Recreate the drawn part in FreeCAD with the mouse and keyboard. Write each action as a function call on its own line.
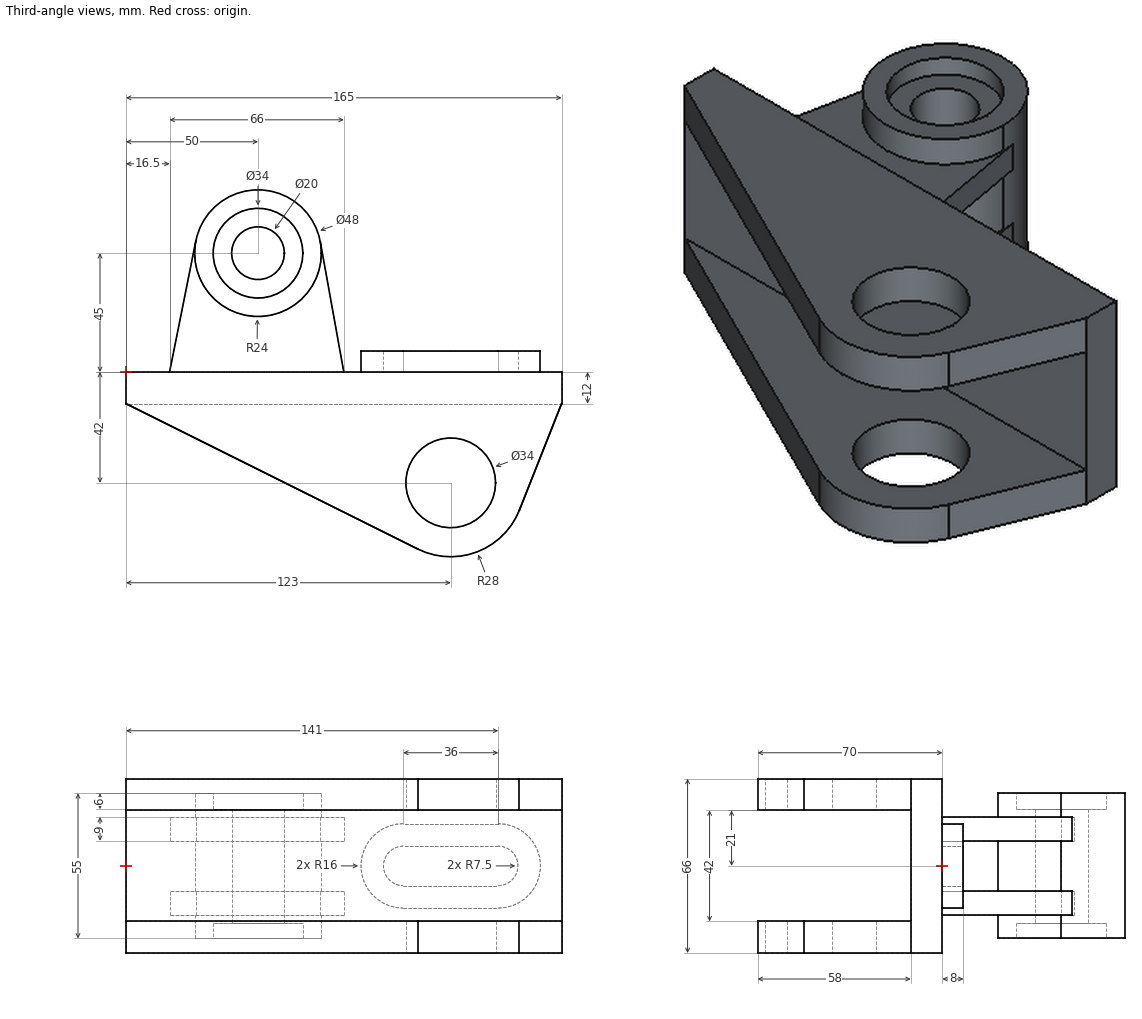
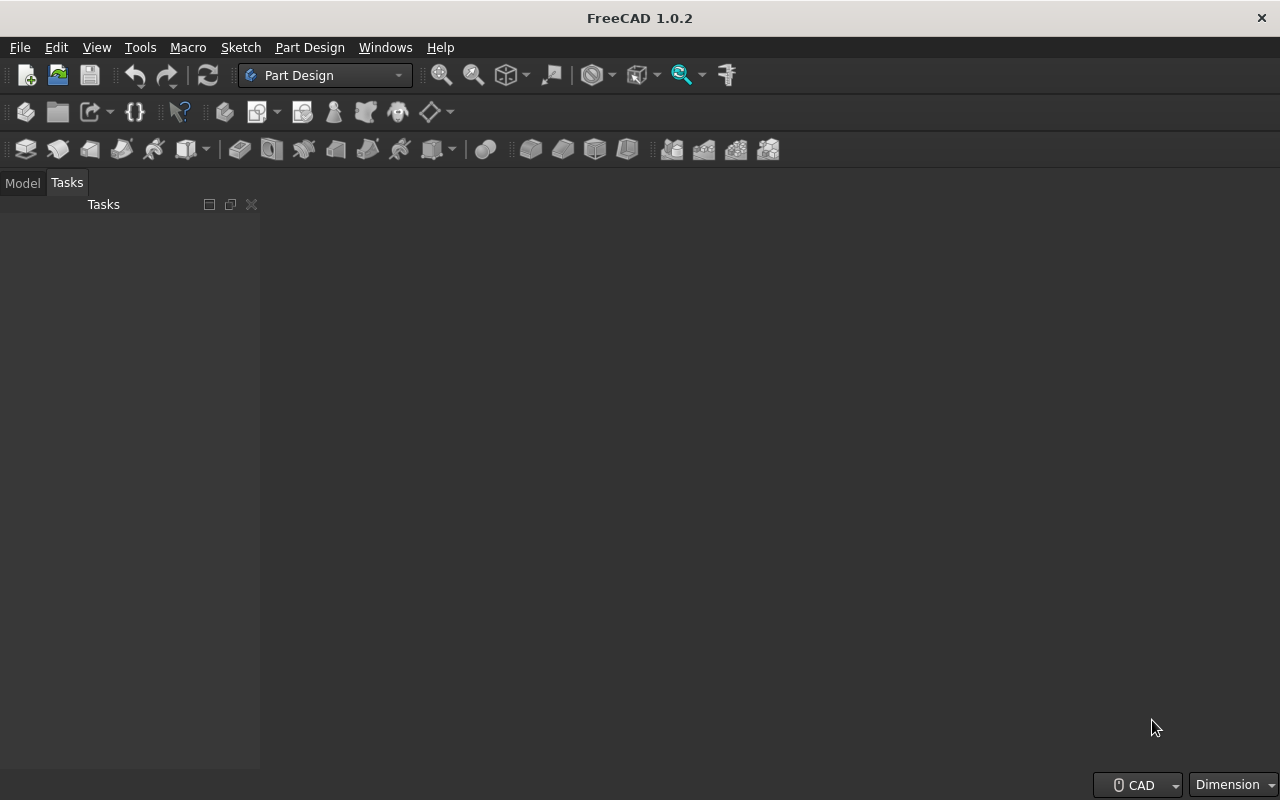
key(ctrl+n)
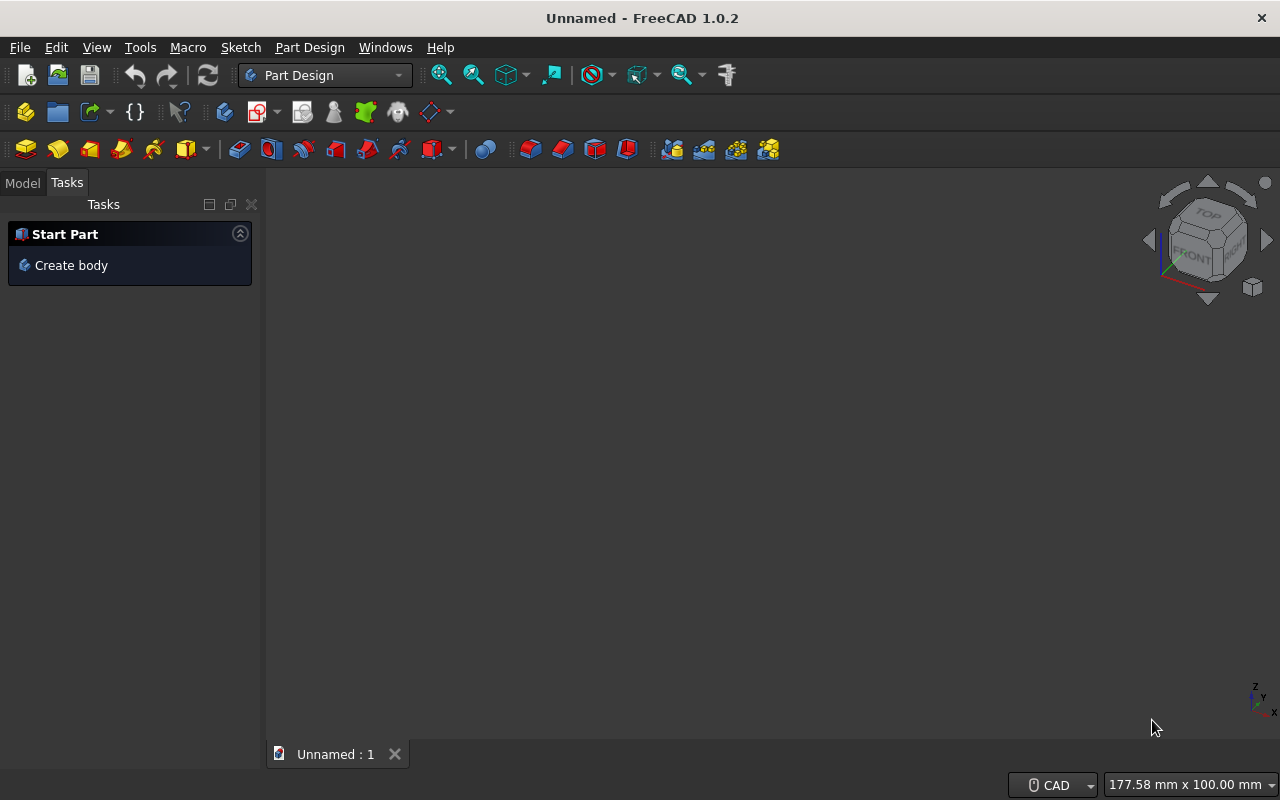
click(258, 112)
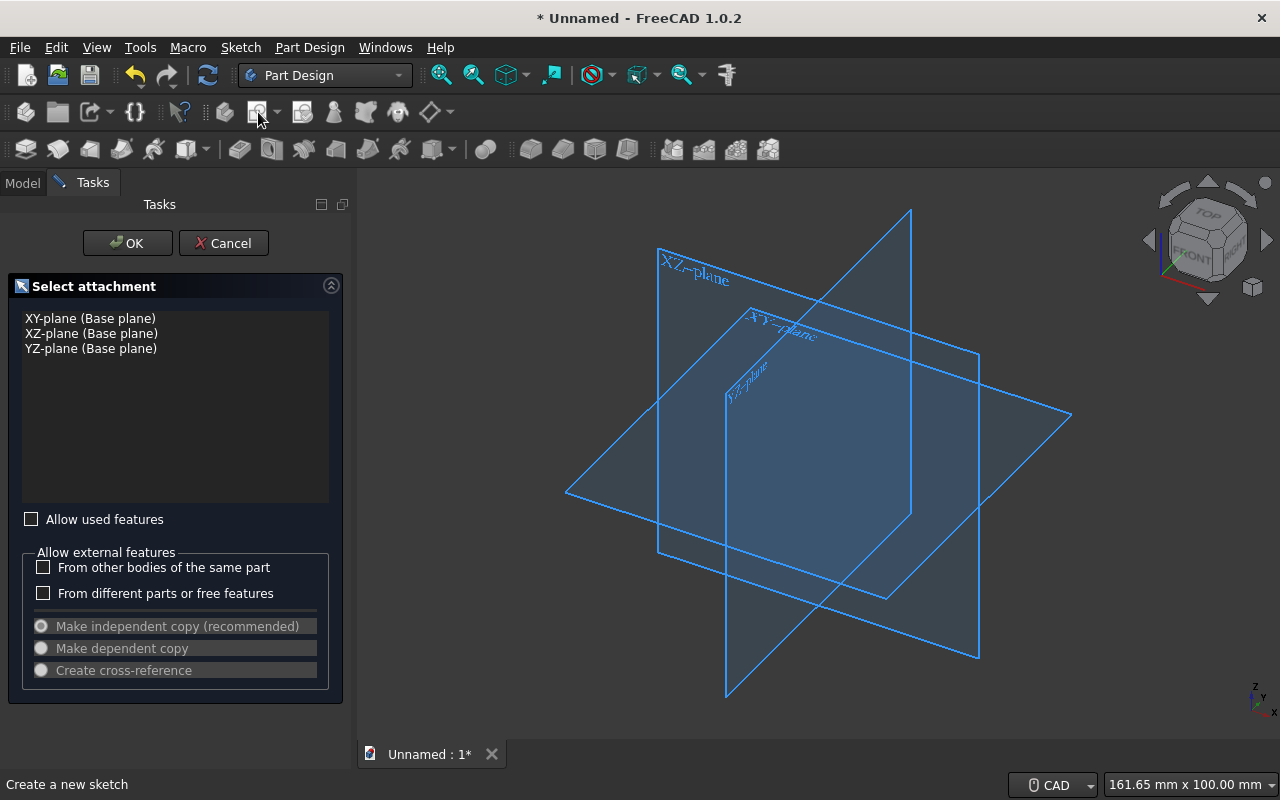
click(82, 318)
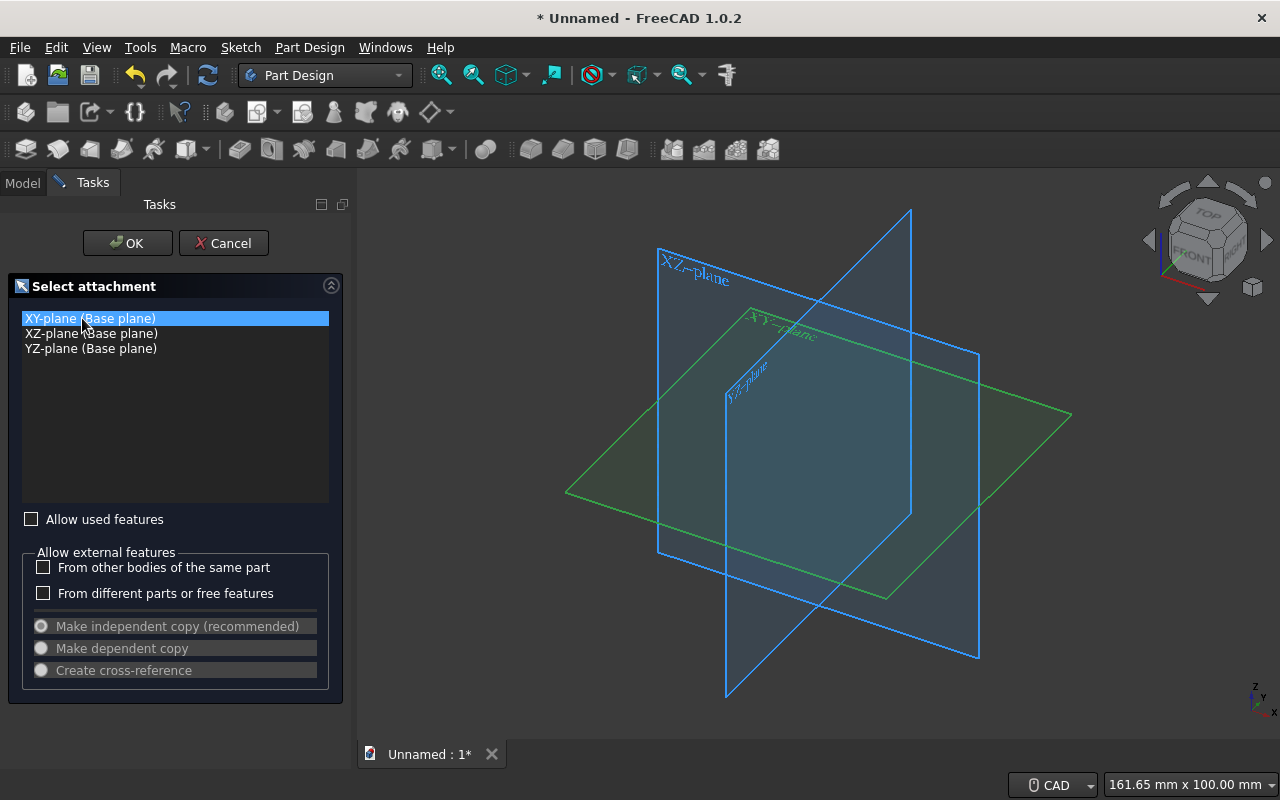
click(128, 243)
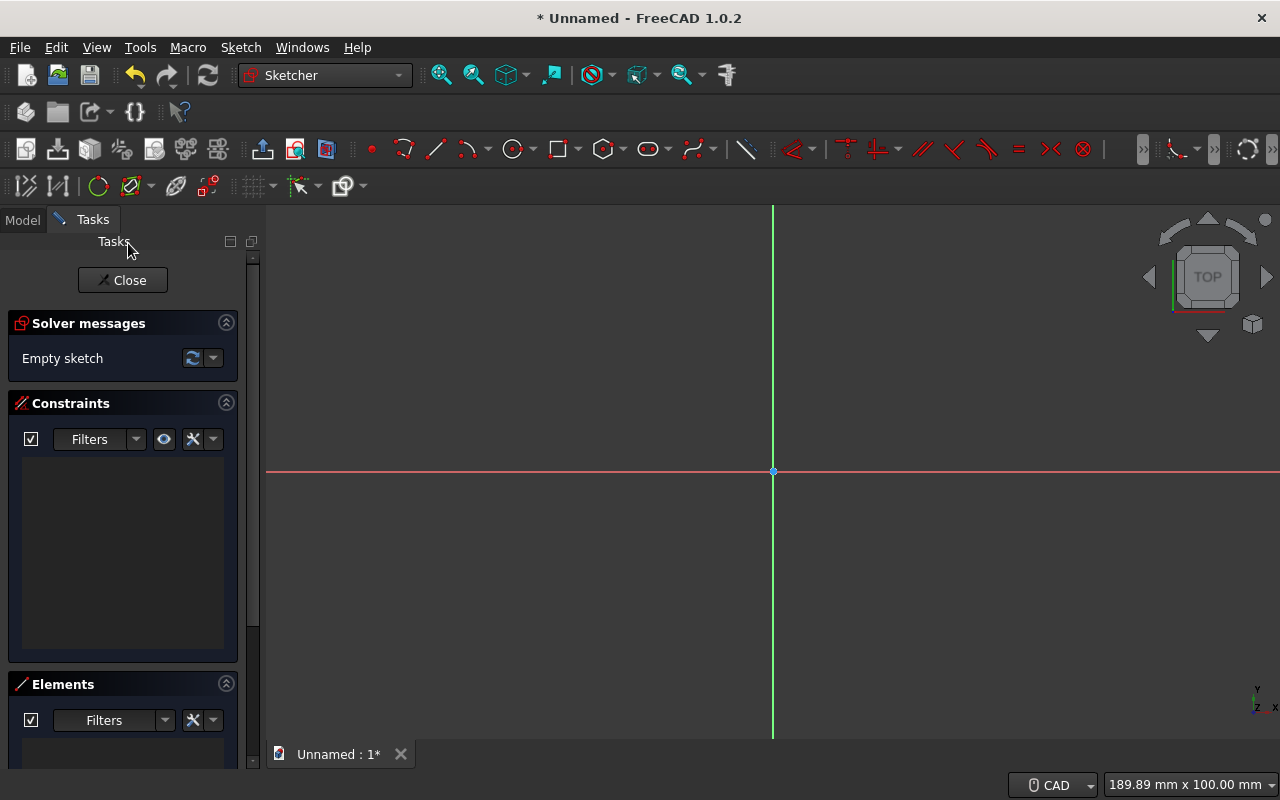
scroll(294, 251, down, 3)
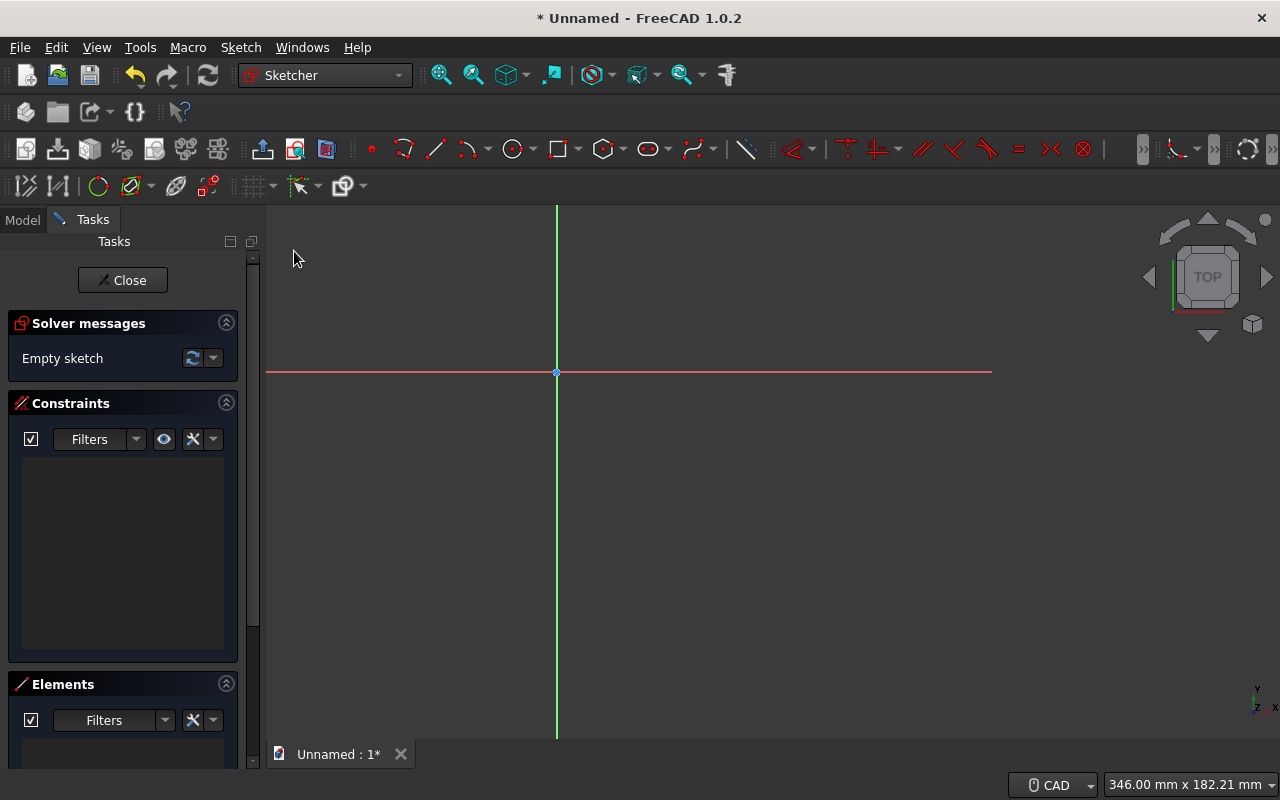
key(g)
key(m)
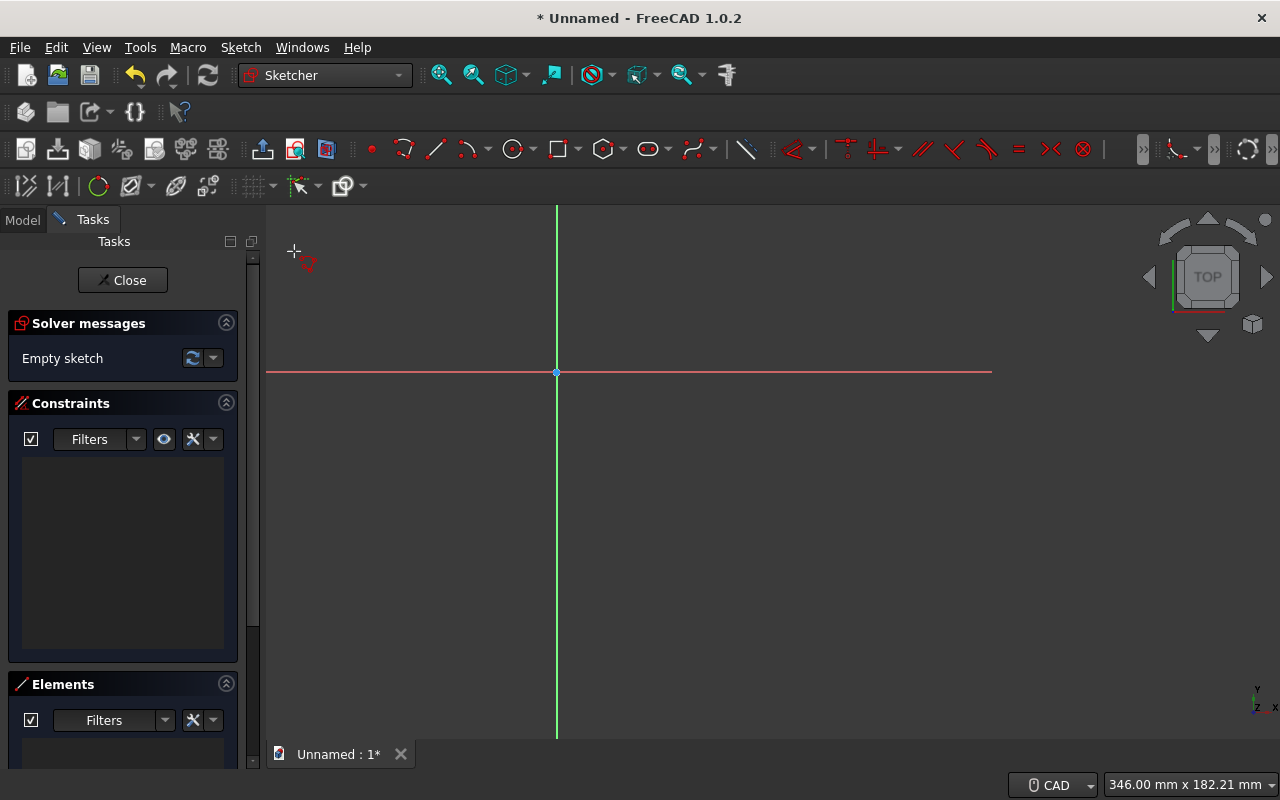
click(994, 526)
click(1040, 407)
click(1040, 372)
click(557, 372)
click(566, 407)
click(881, 569)
right_click(881, 569)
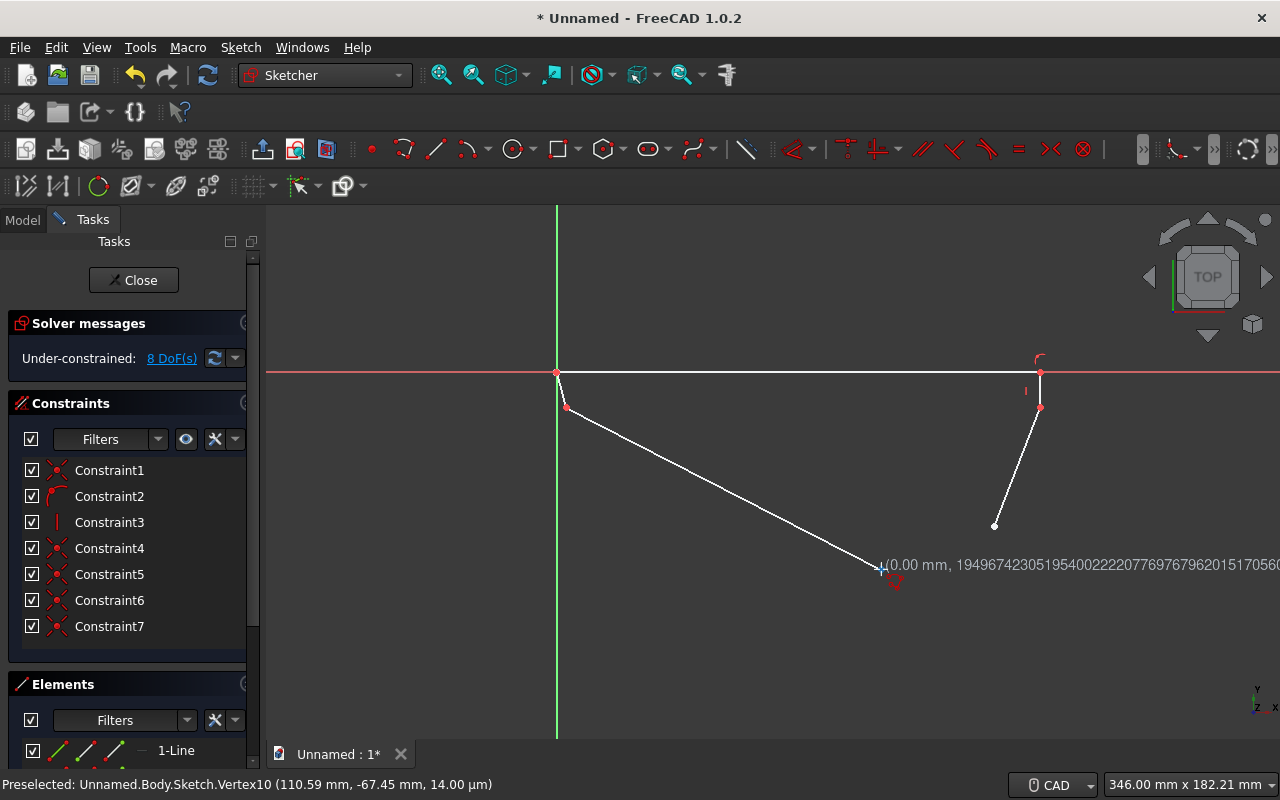
key(g)
key(3)
key(a)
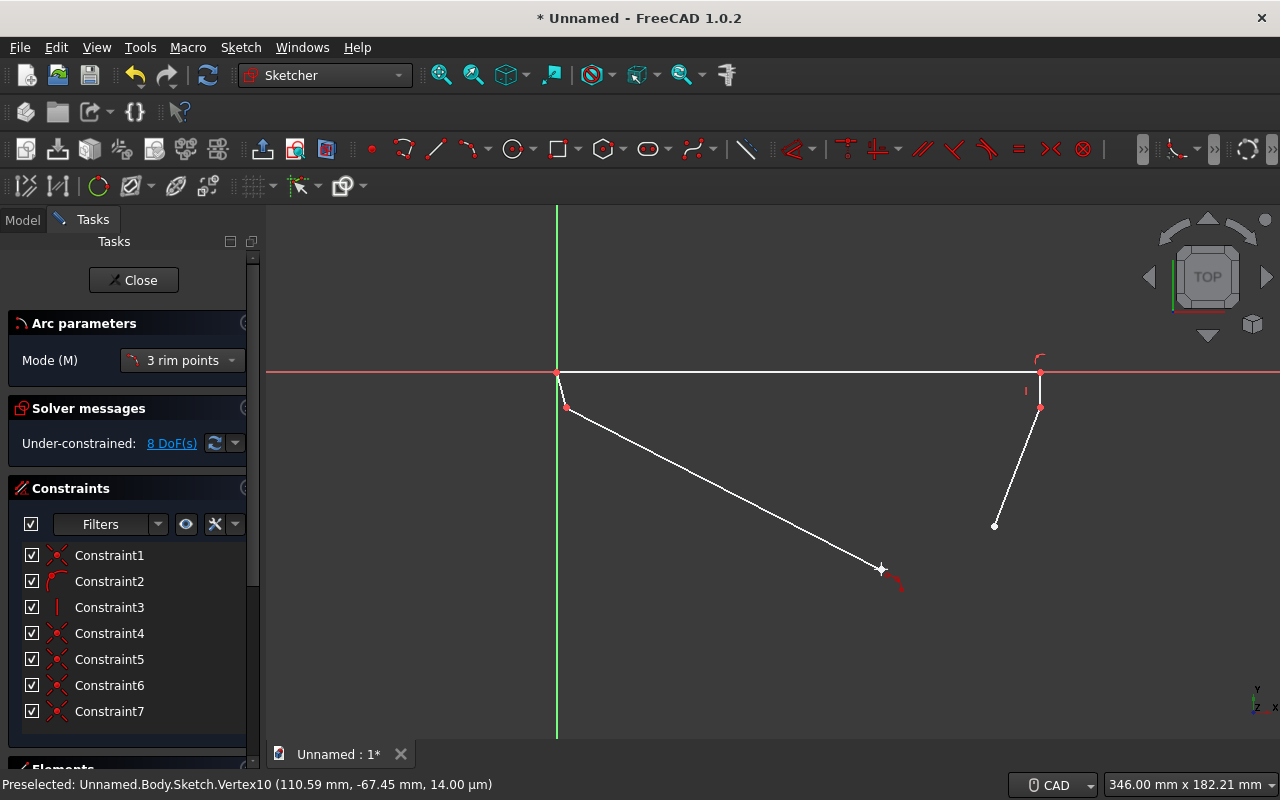
click(881, 570)
click(994, 527)
click(947, 572)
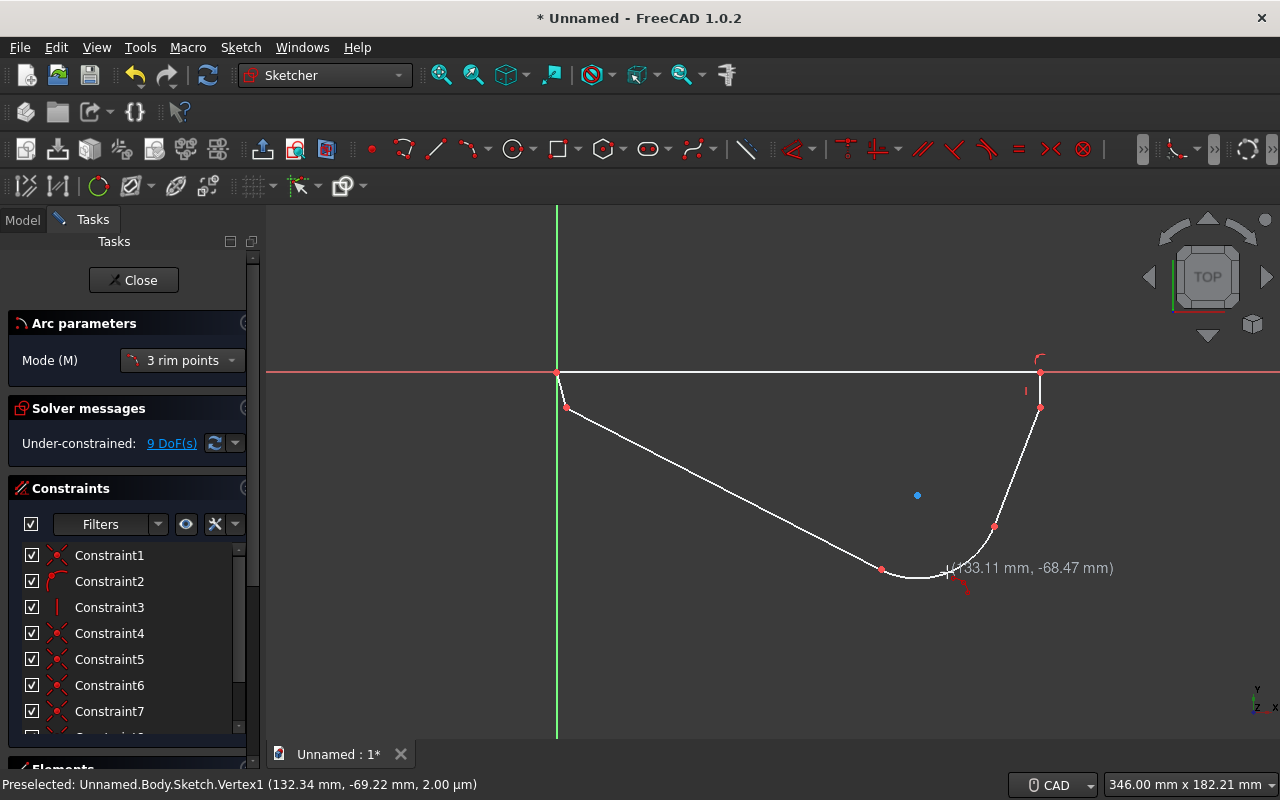
key(g)
key(c)